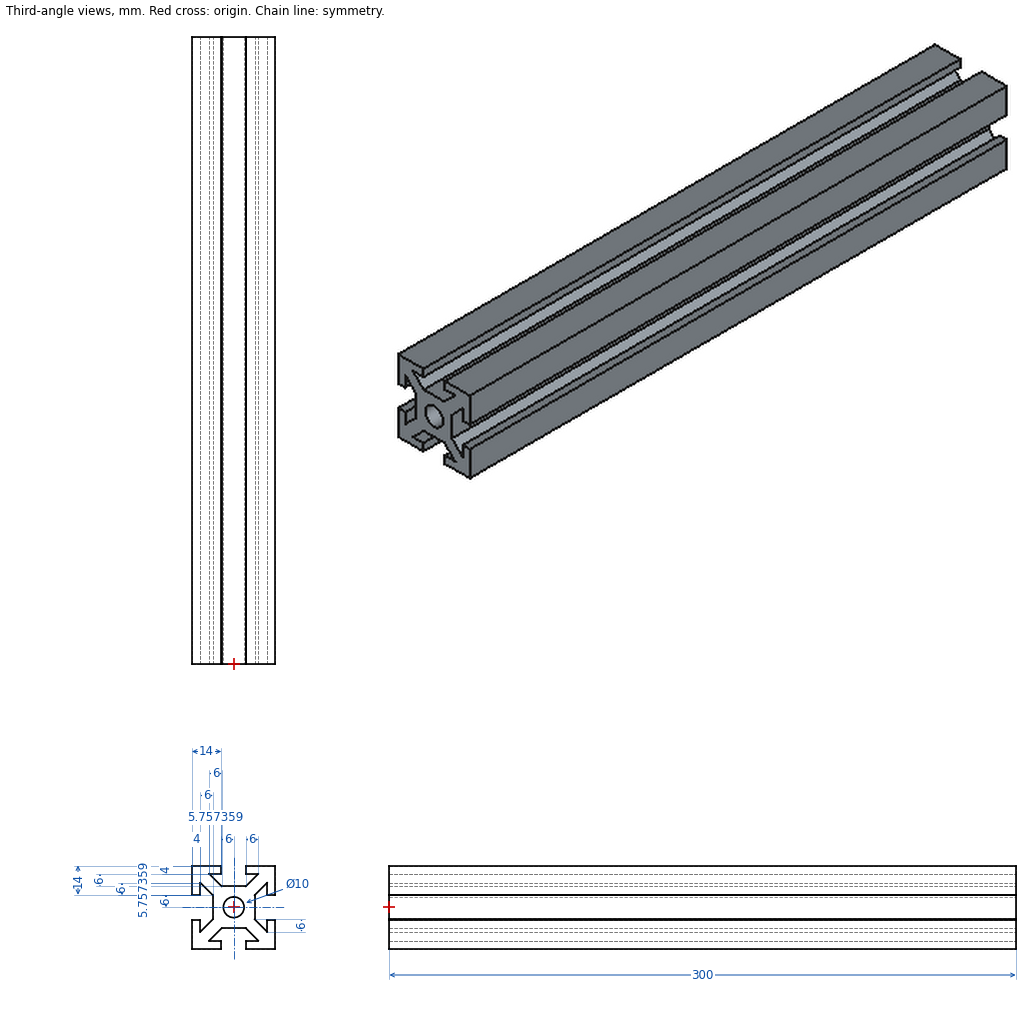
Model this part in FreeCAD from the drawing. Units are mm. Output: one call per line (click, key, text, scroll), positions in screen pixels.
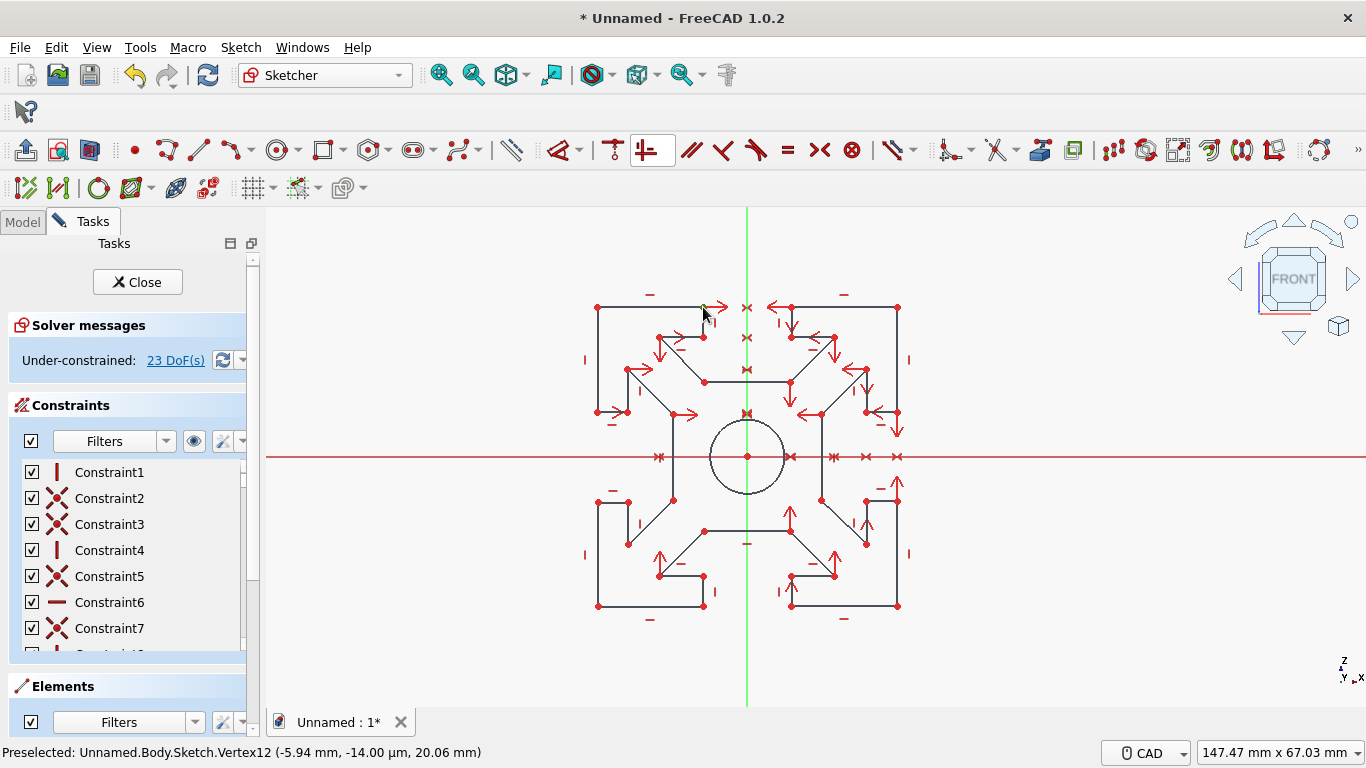
click(703, 607)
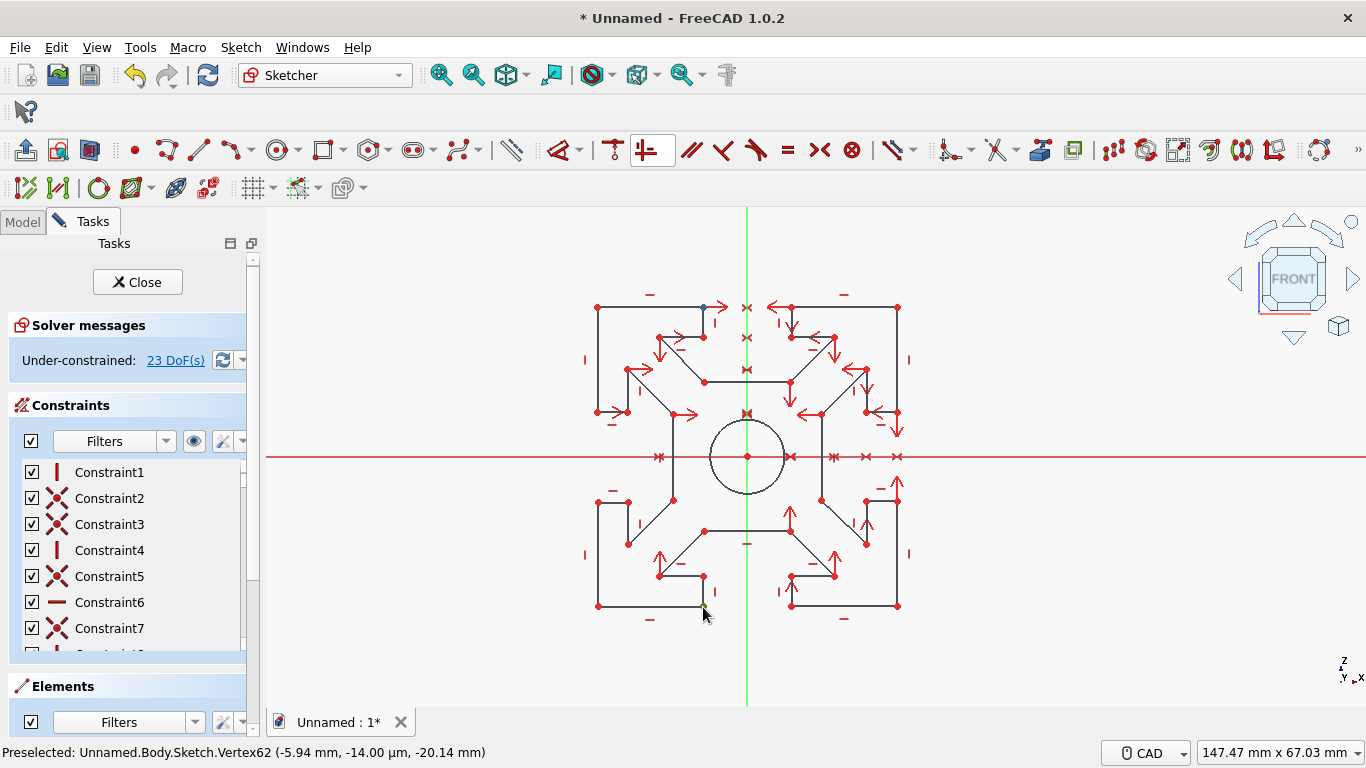
click(359, 457)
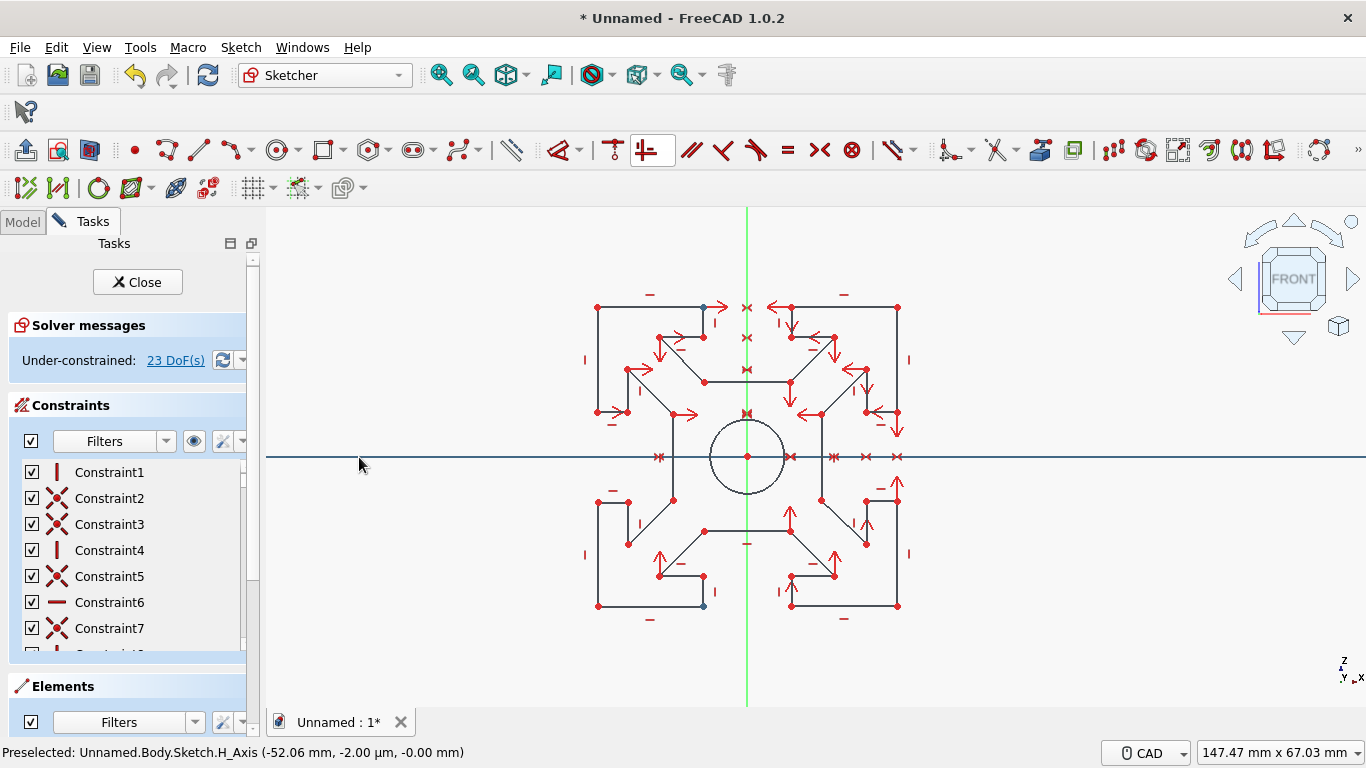
key(s)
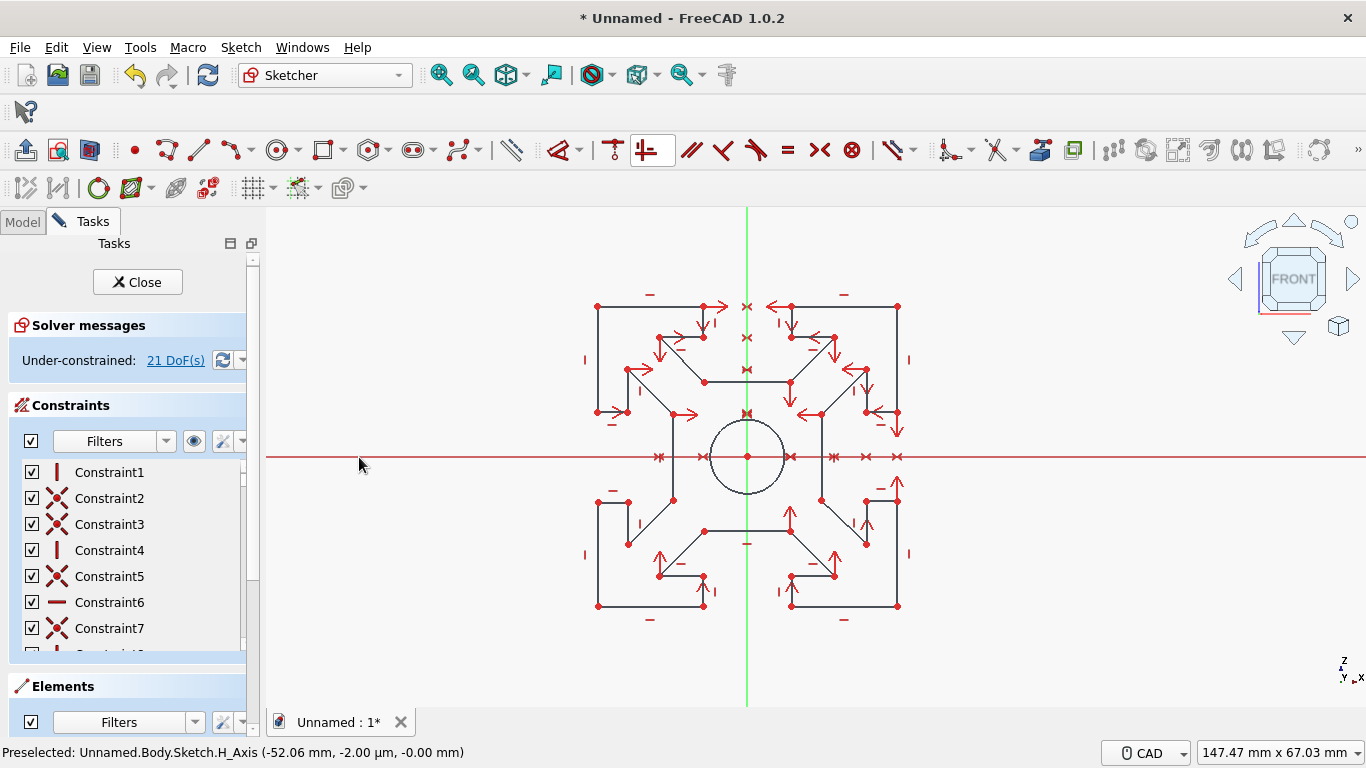
click(598, 412)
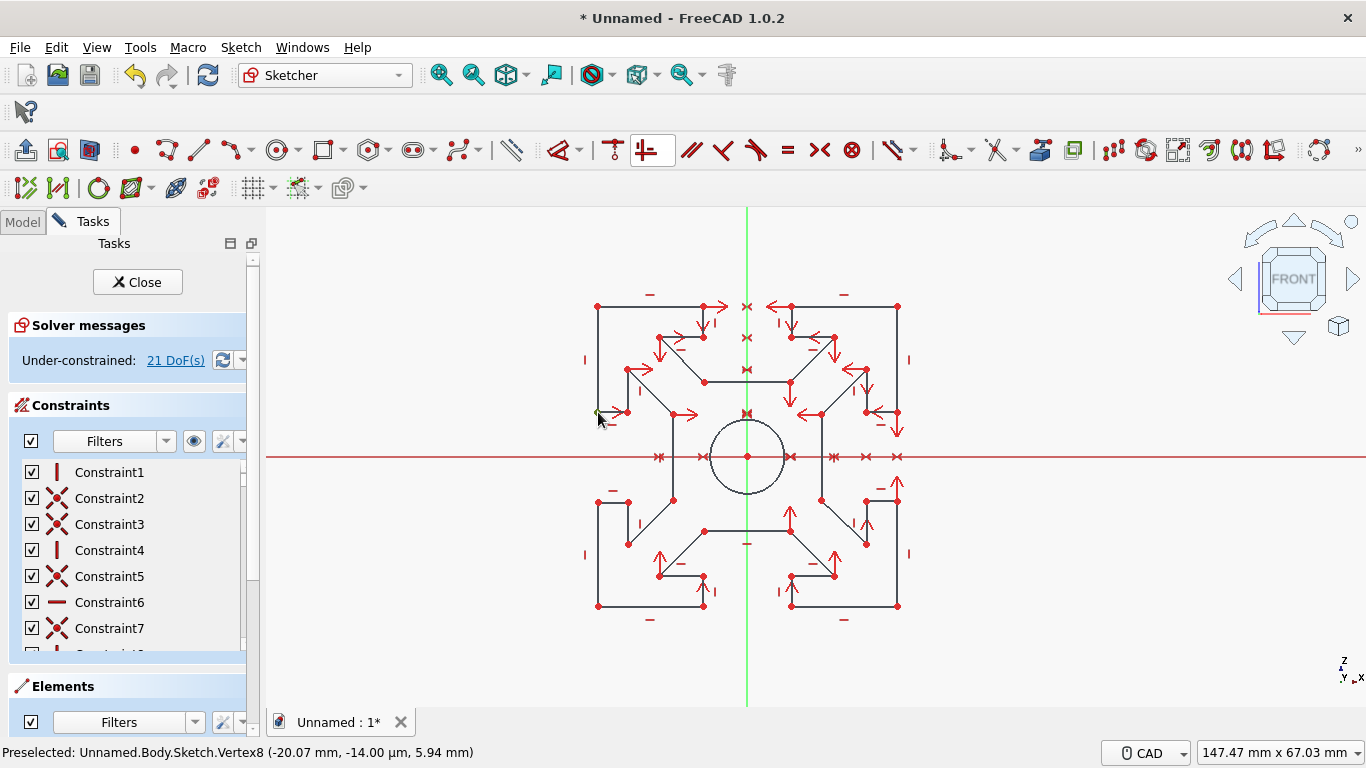
click(598, 503)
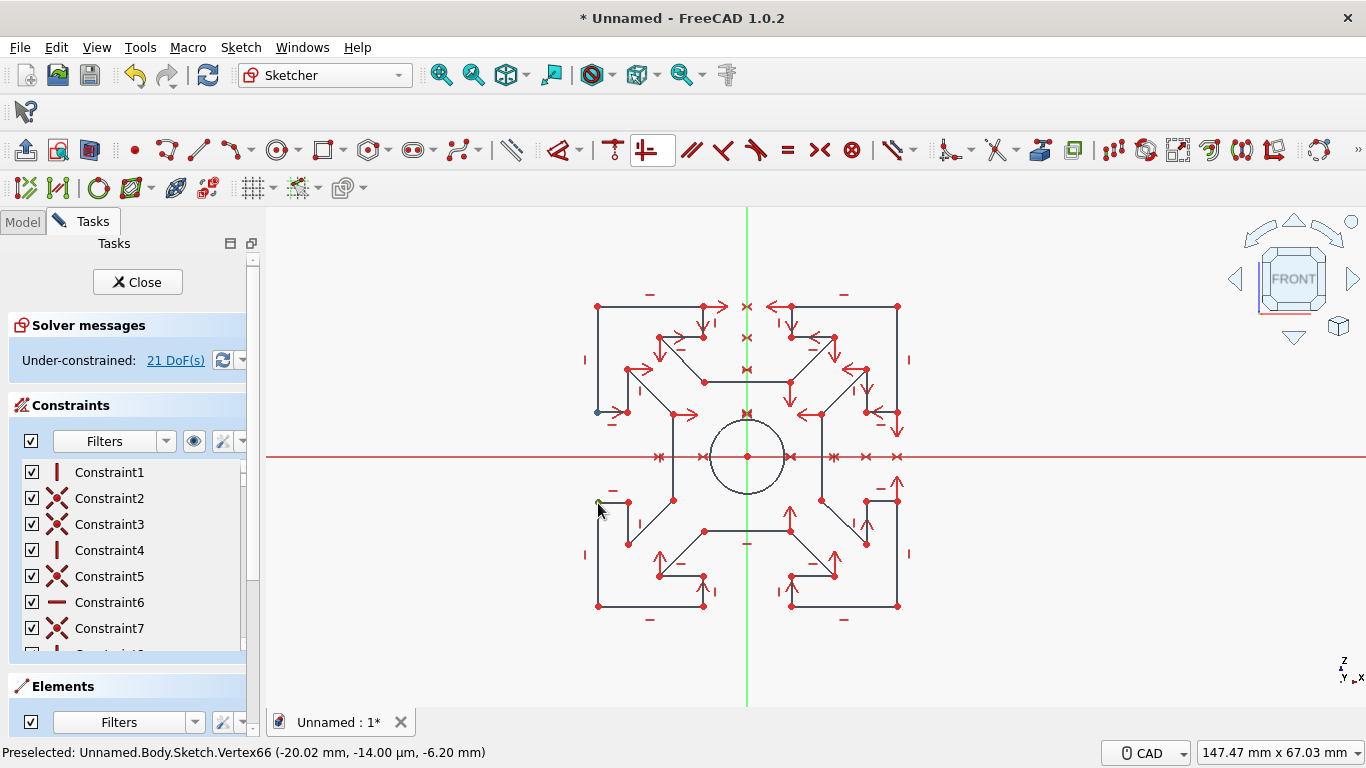
click(359, 457)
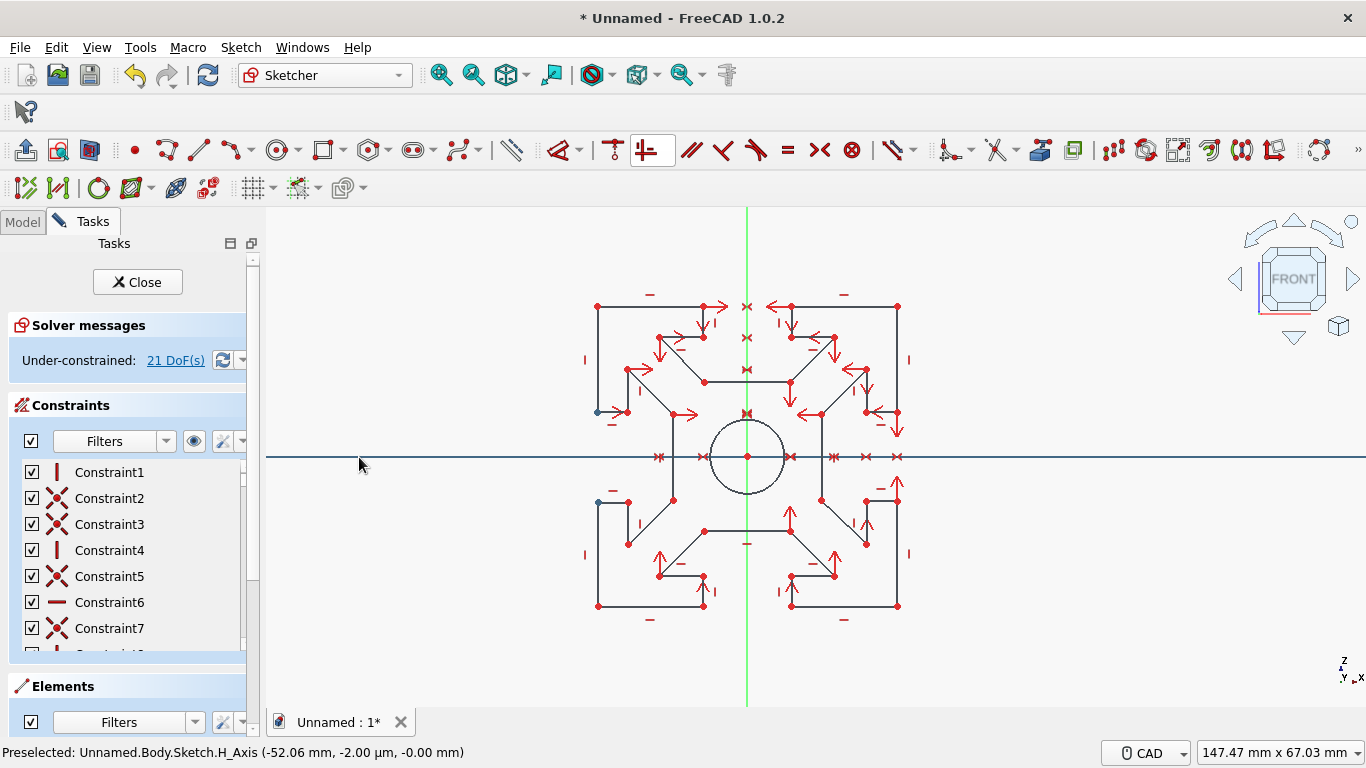
click(820, 150)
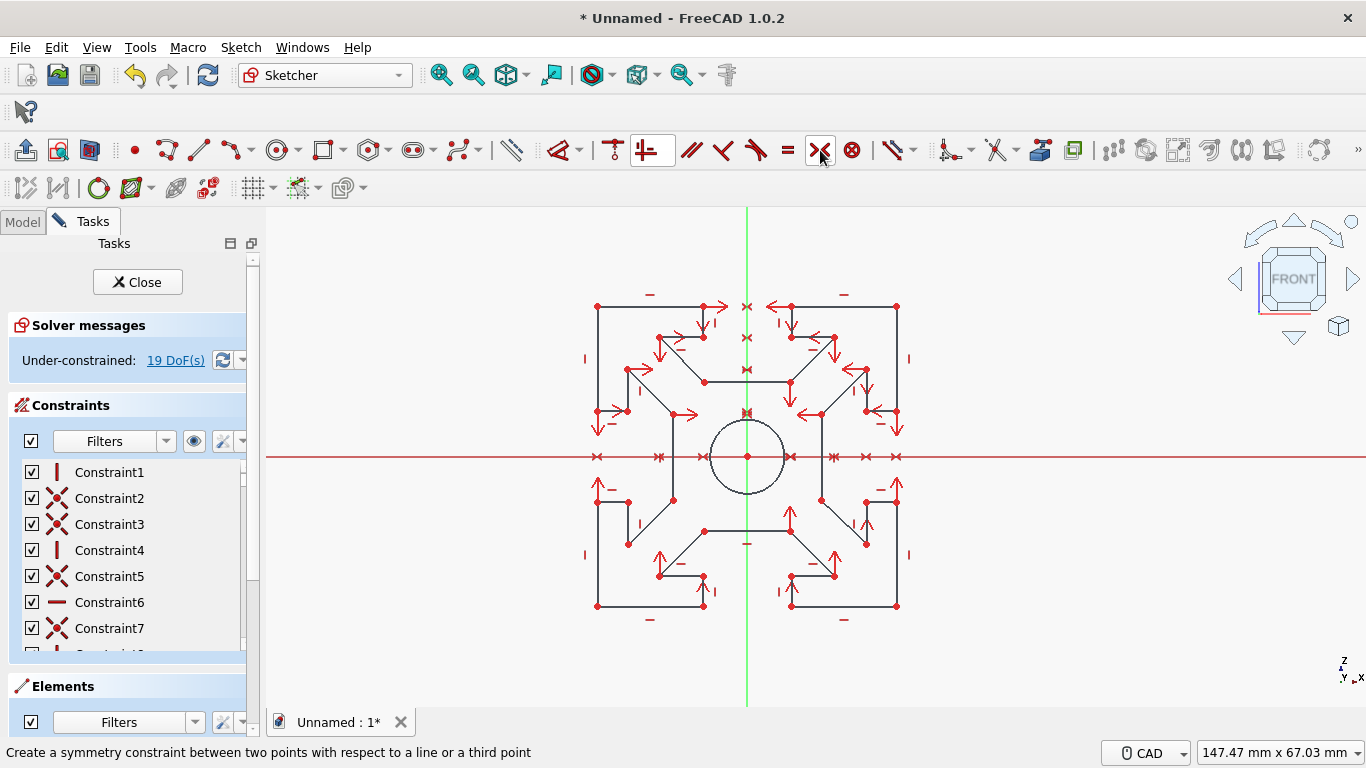
click(628, 369)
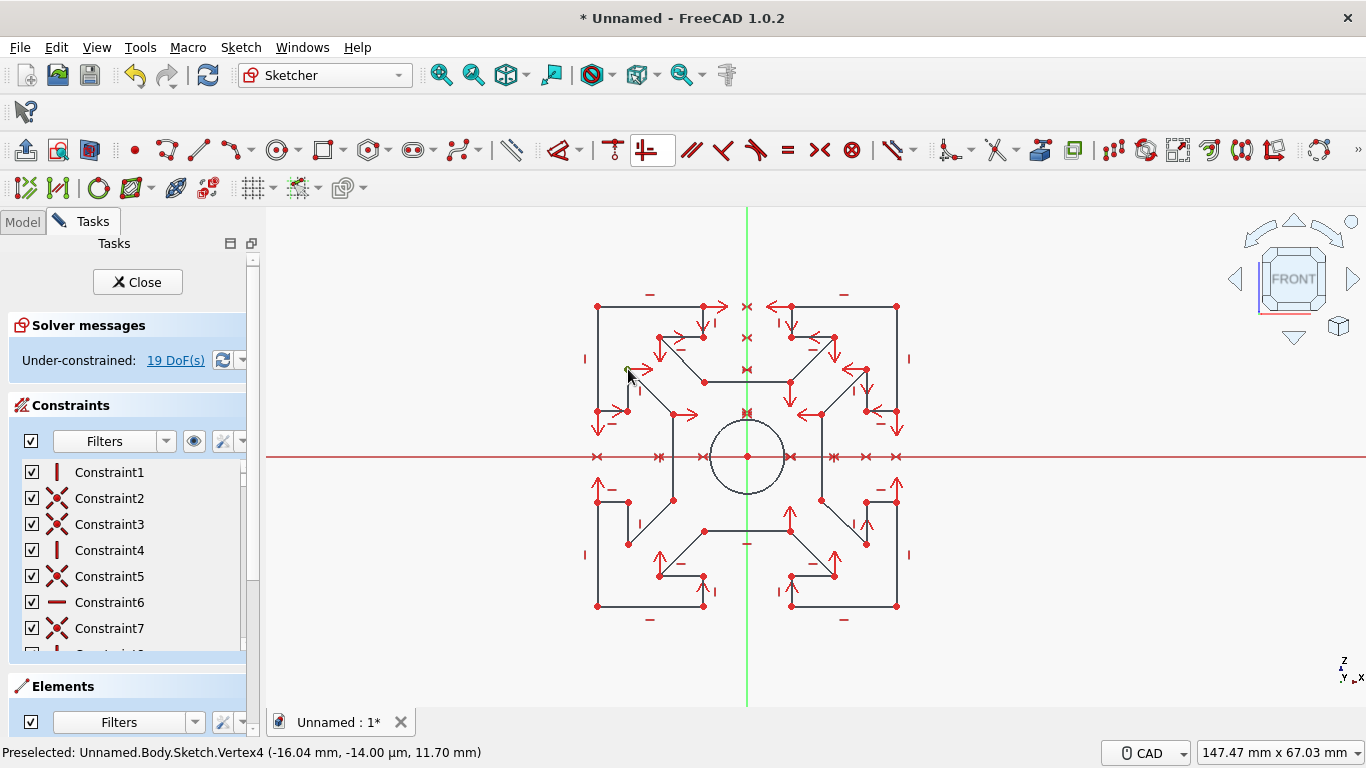
click(628, 545)